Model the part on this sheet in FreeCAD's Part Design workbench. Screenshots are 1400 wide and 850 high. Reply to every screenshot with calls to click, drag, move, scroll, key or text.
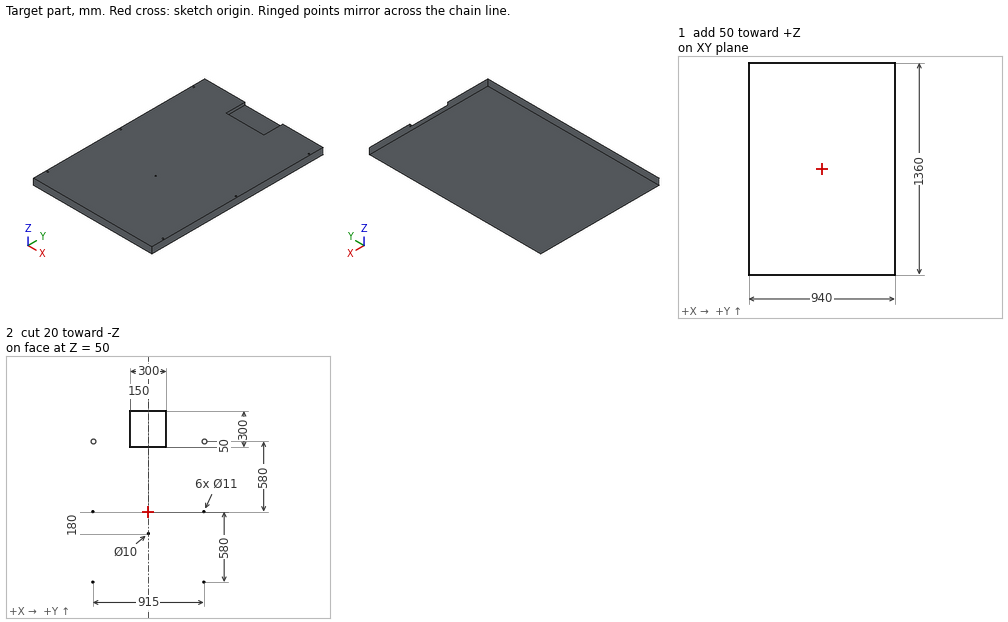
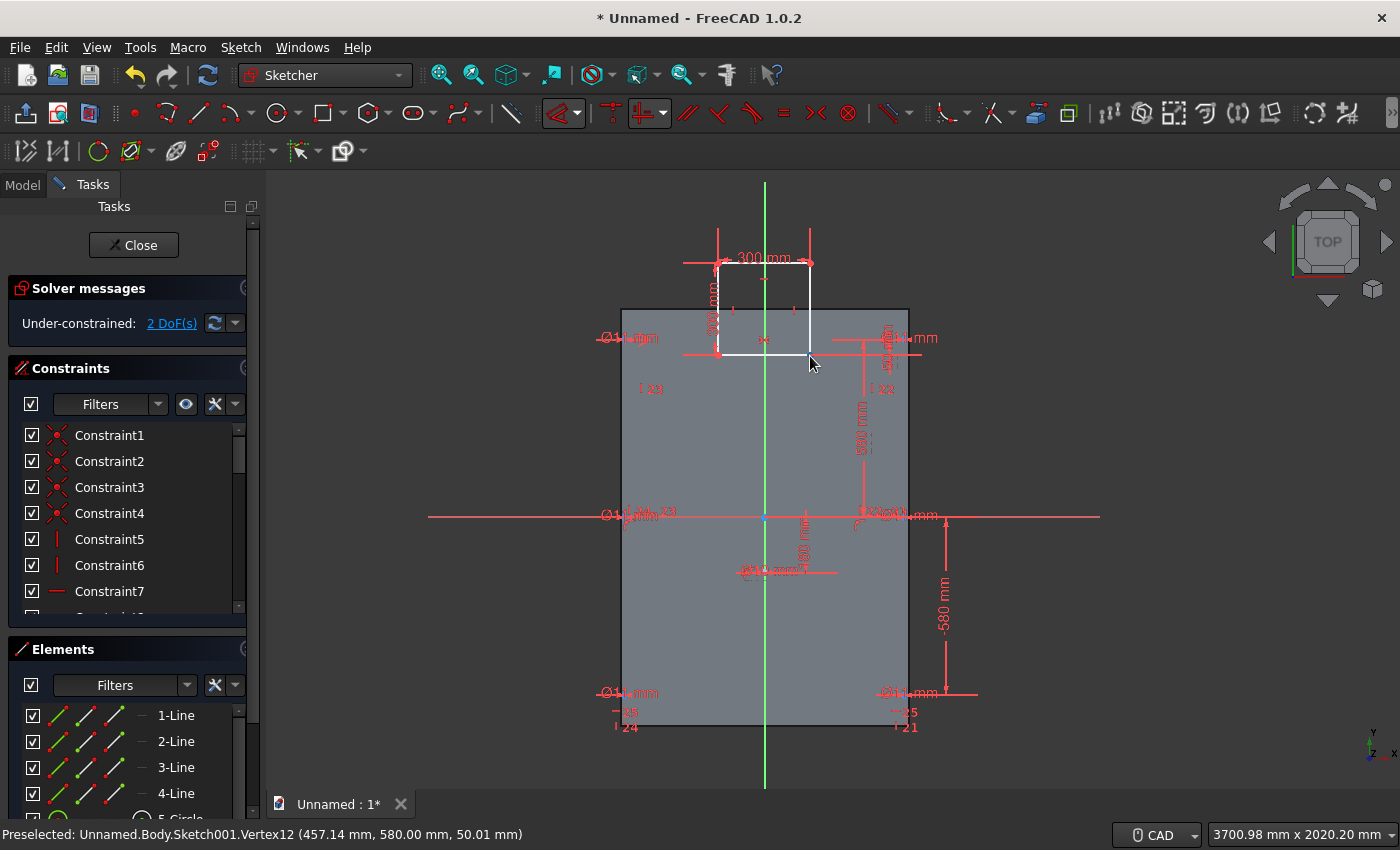
click(718, 263)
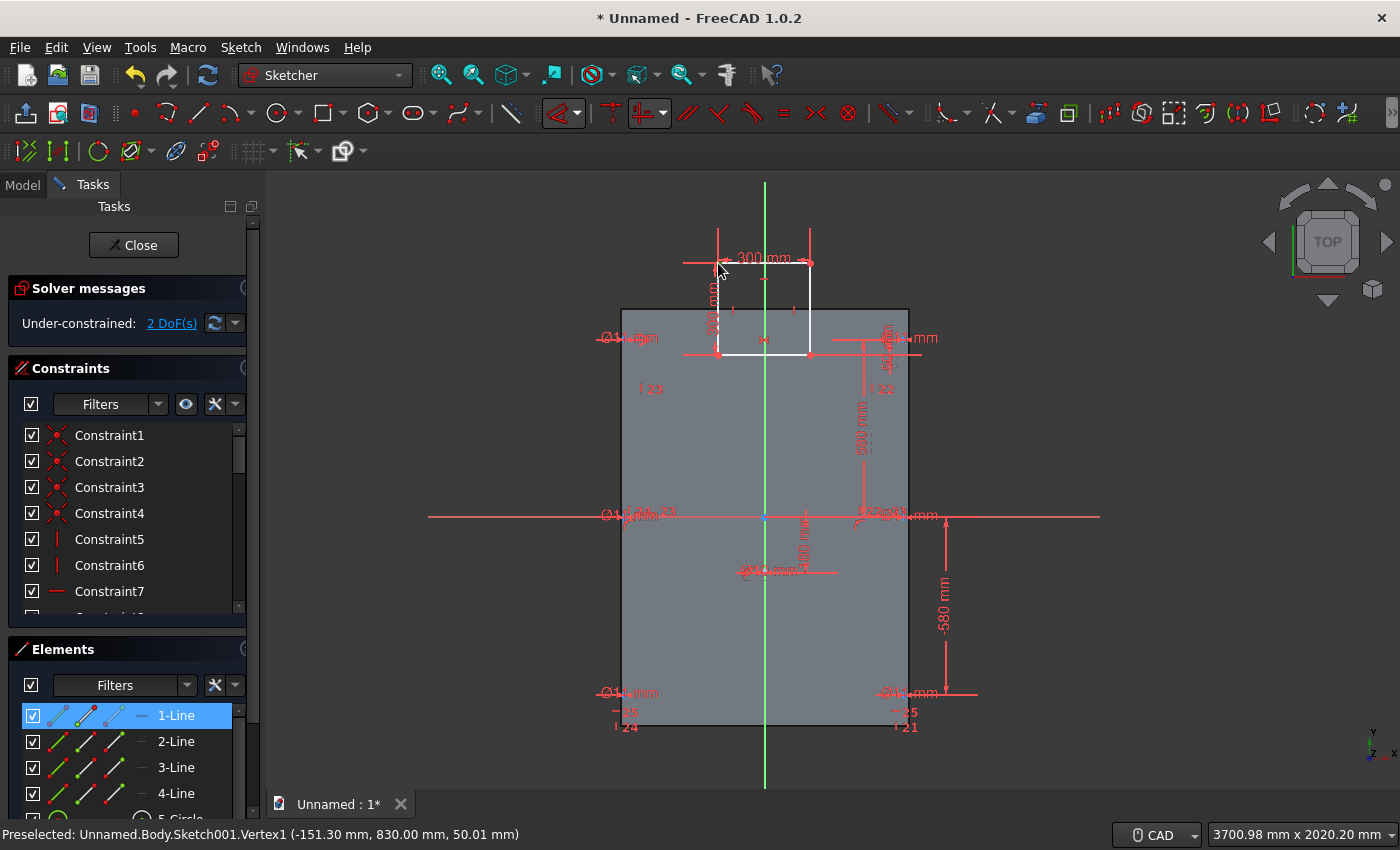
key(l)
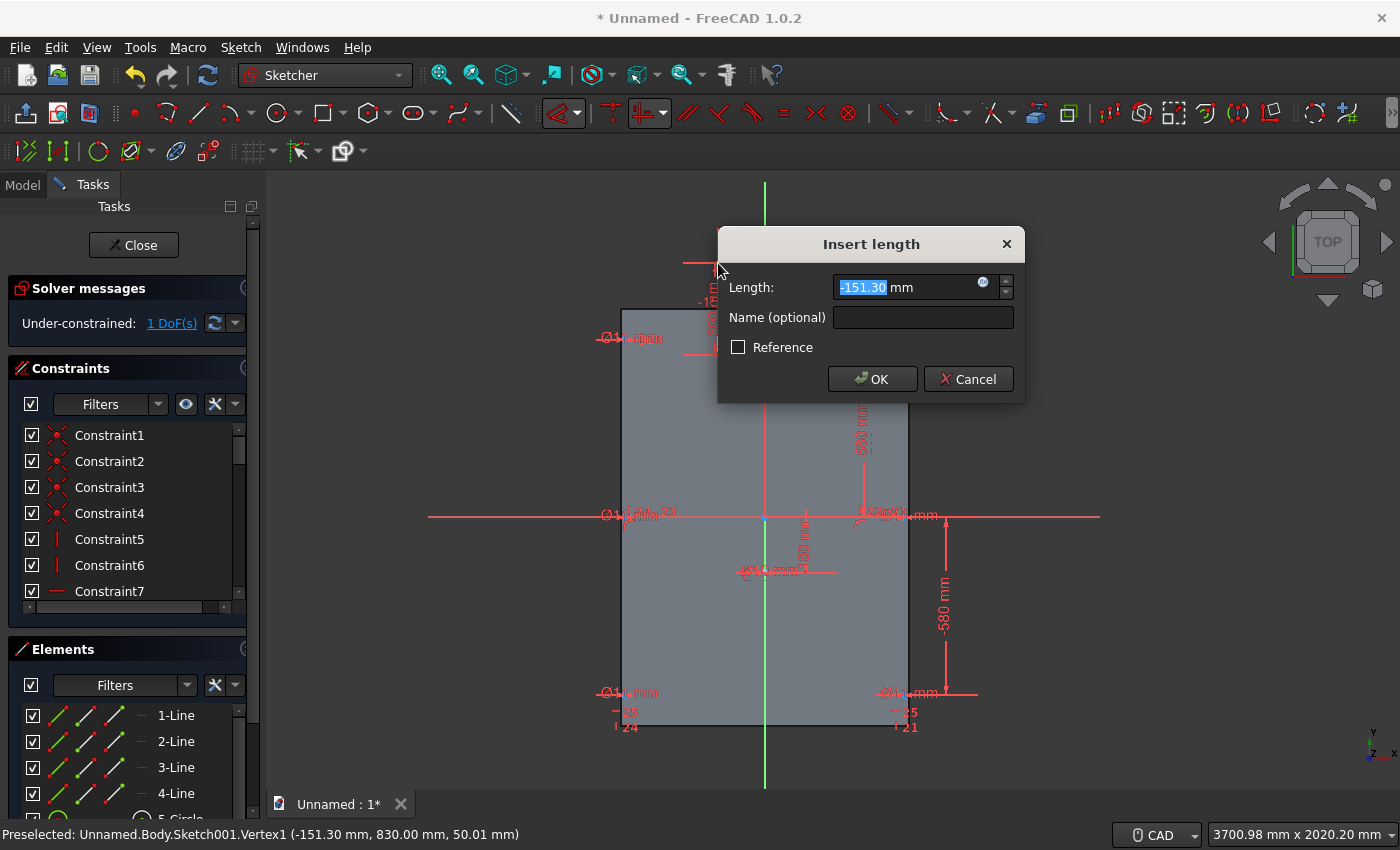
text(-150)
key(Return)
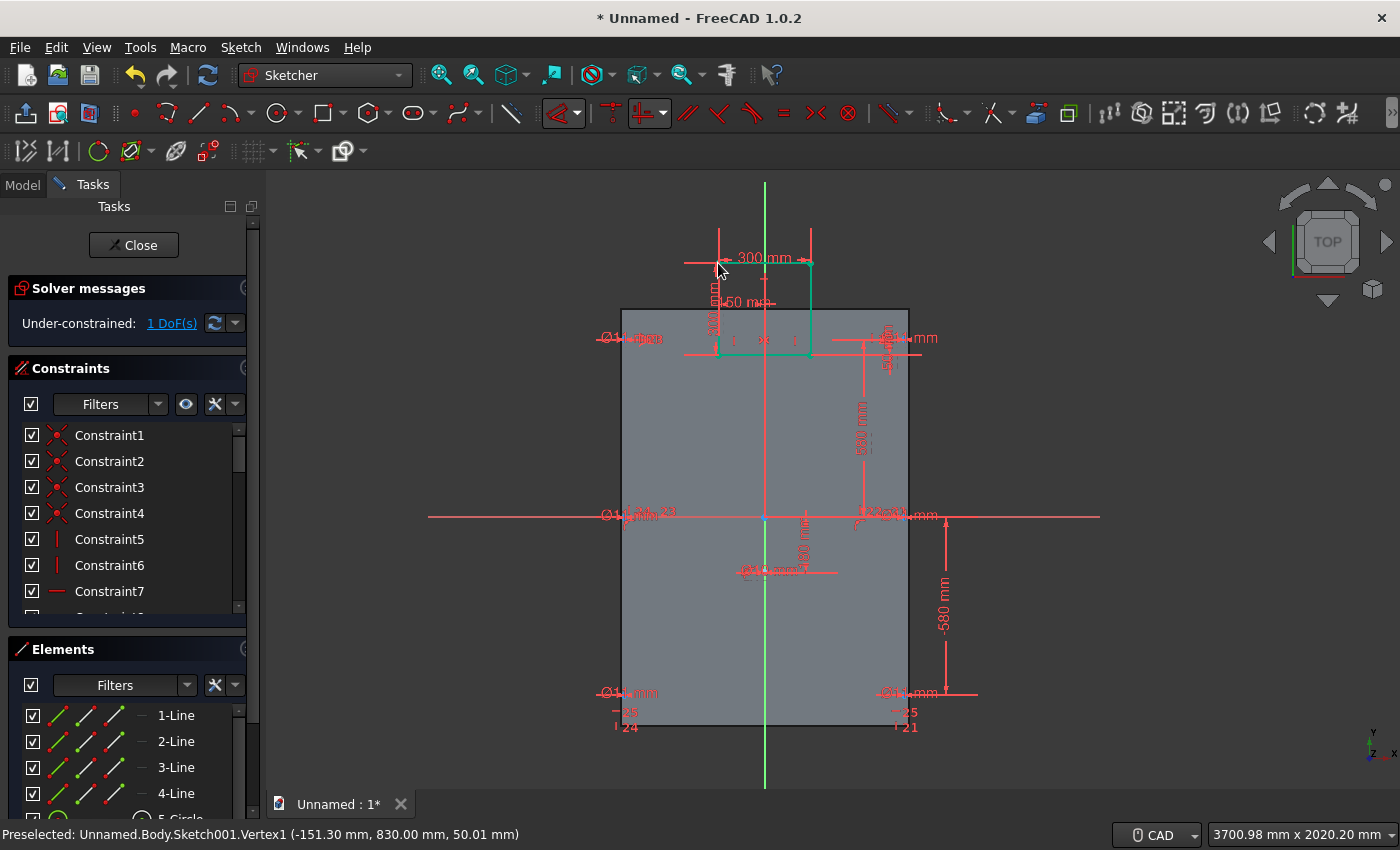
click(905, 695)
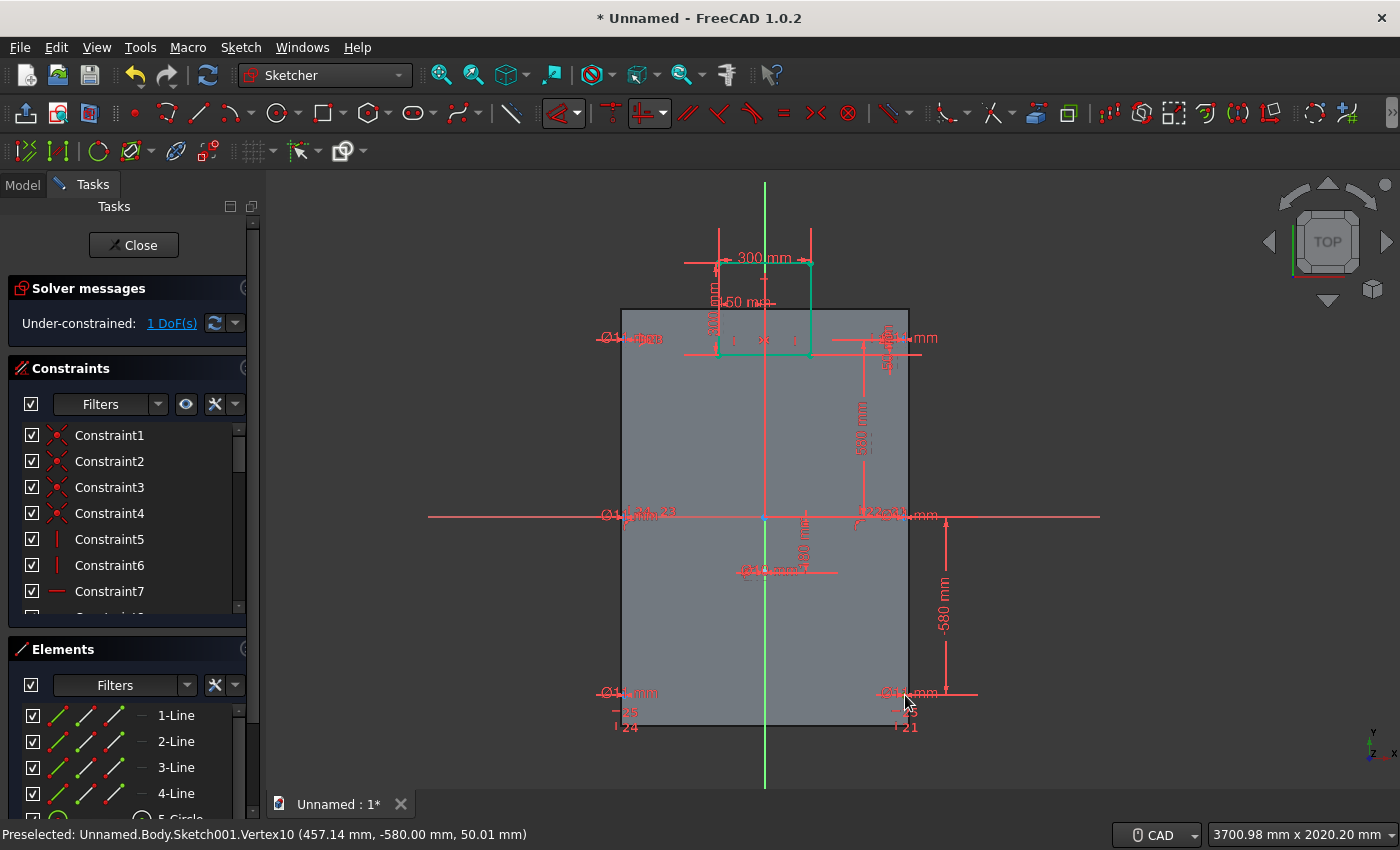
click(625, 695)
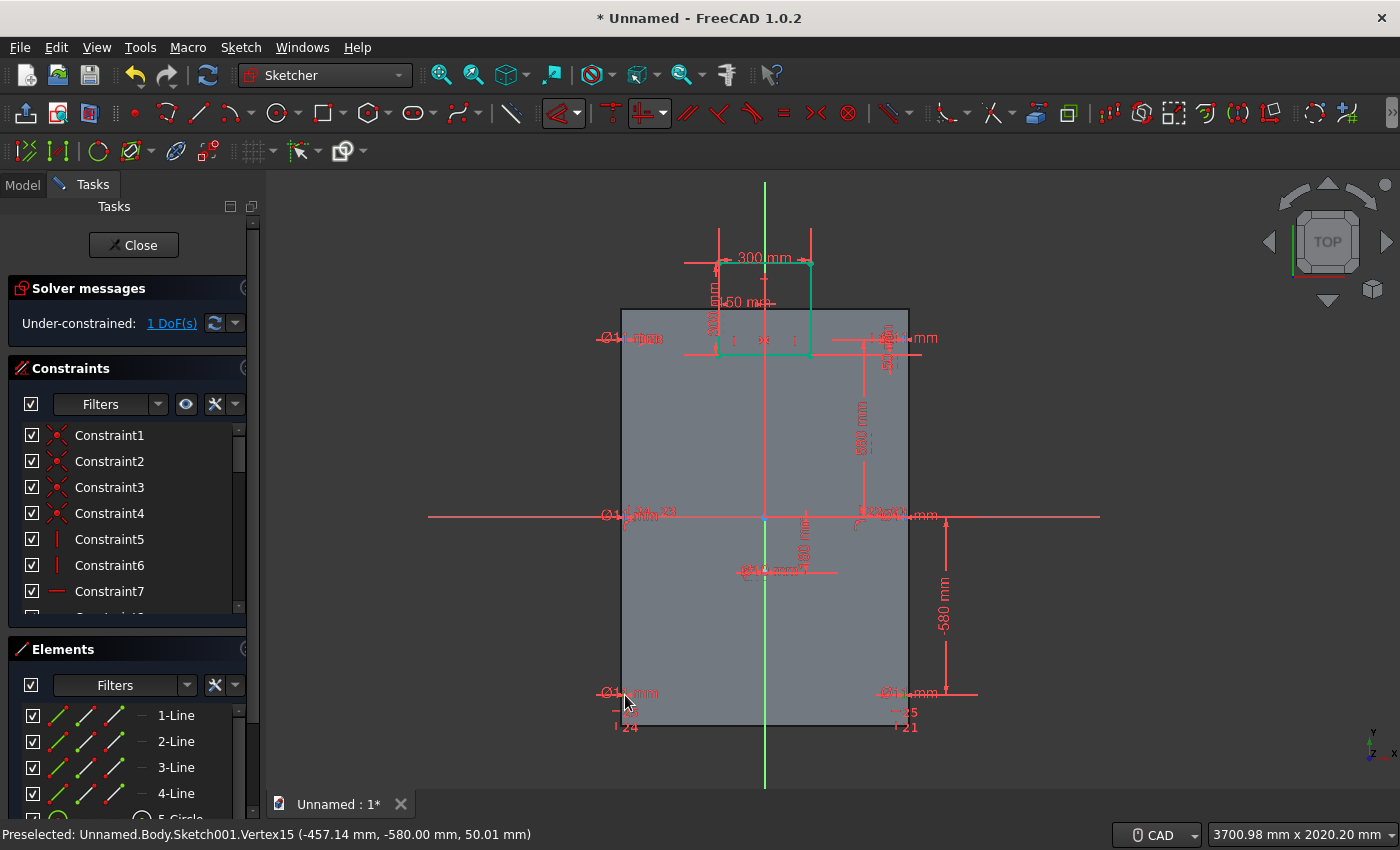
key(l)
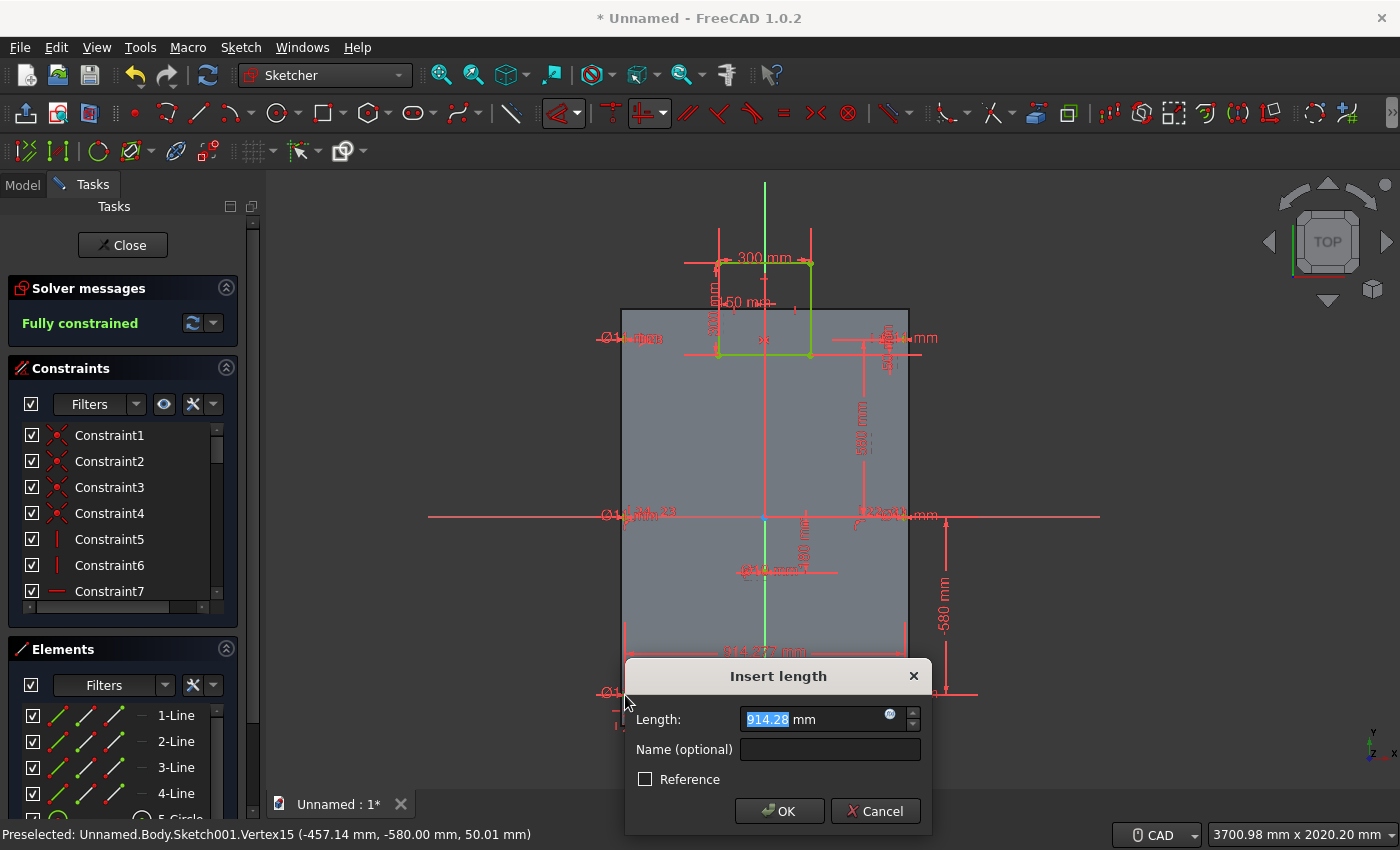
text(915)
key(Return)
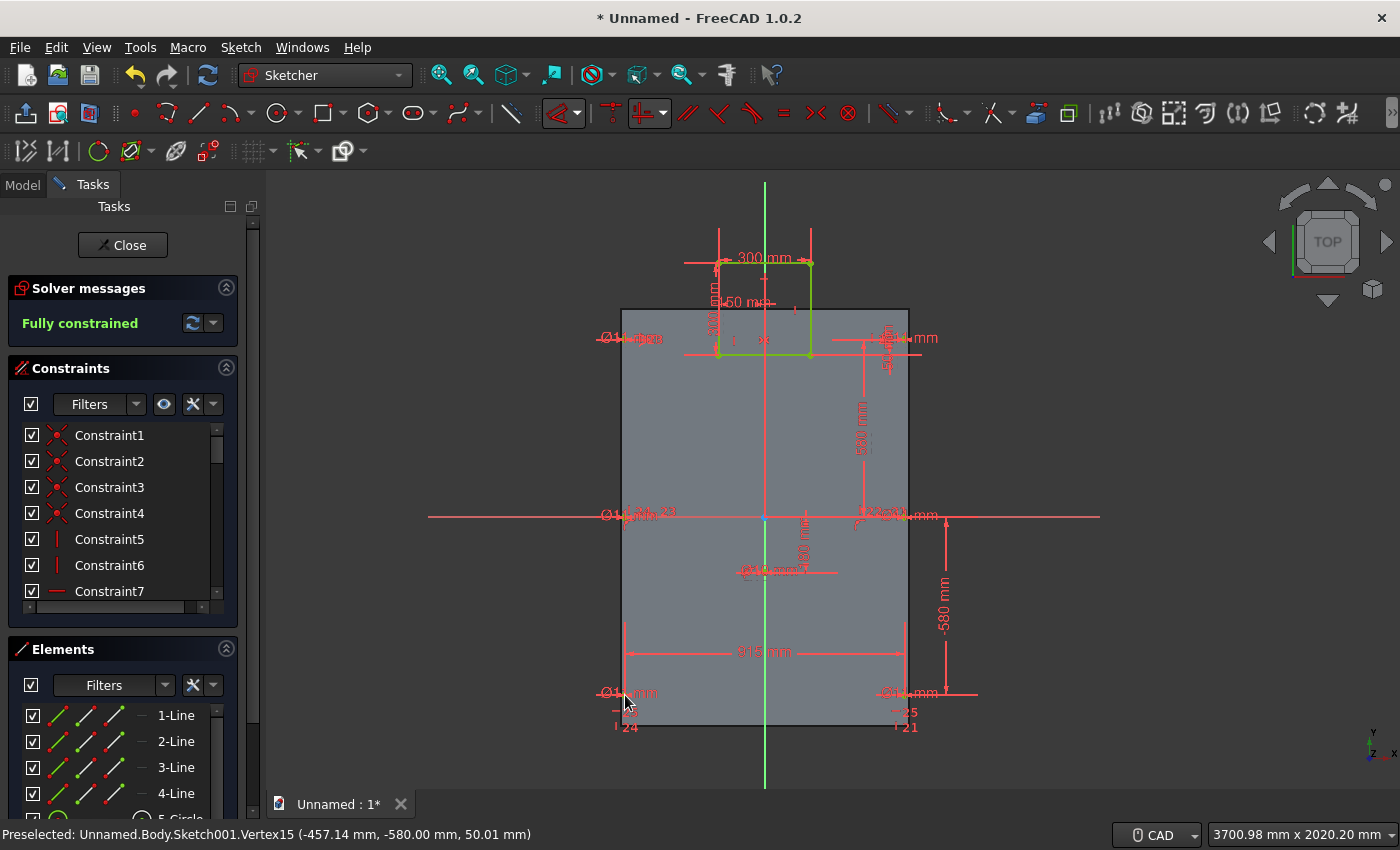
click(123, 245)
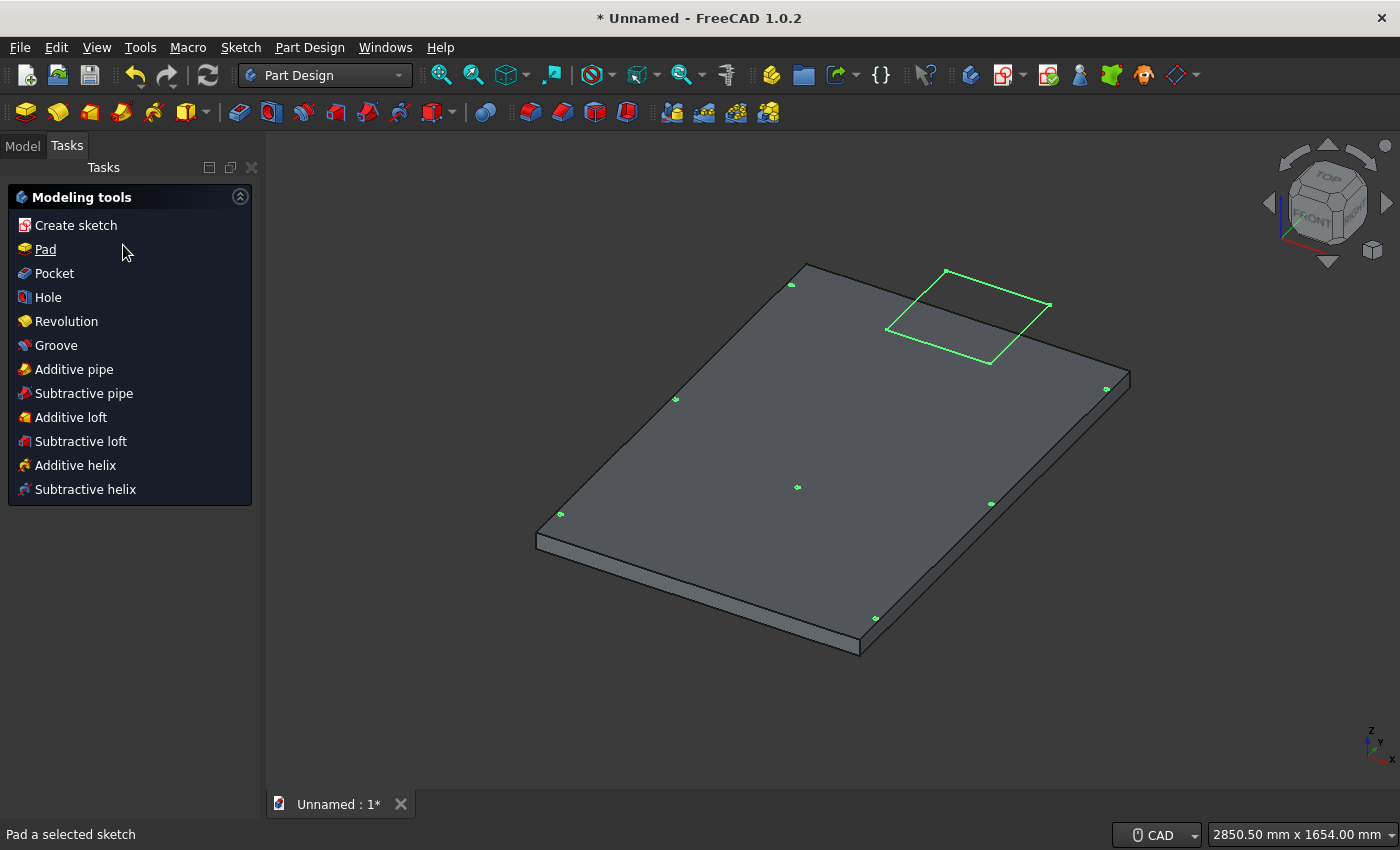
click(240, 112)